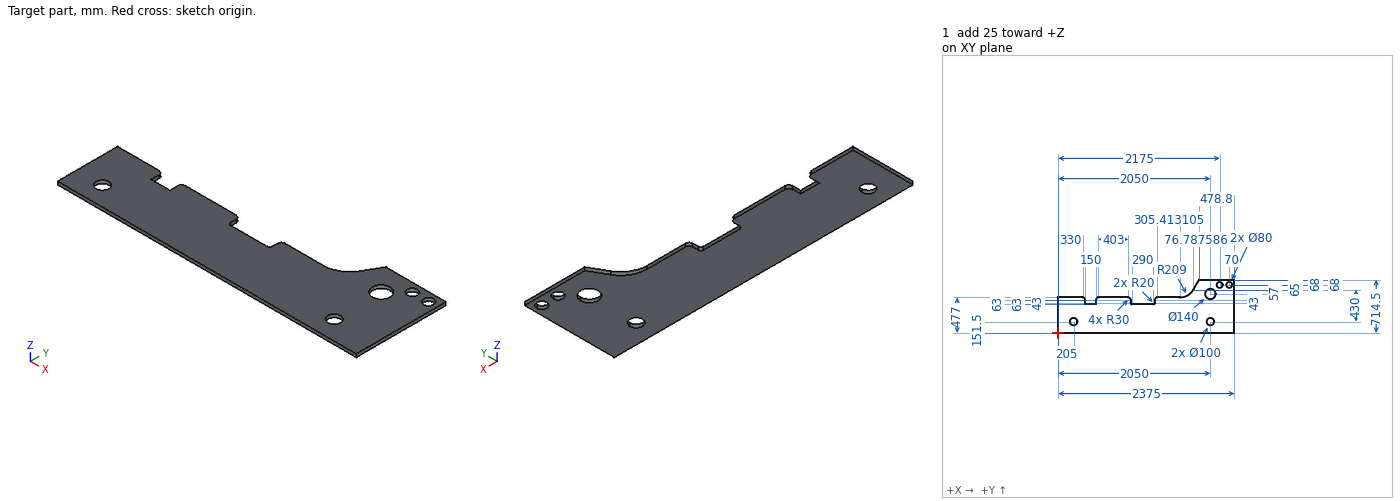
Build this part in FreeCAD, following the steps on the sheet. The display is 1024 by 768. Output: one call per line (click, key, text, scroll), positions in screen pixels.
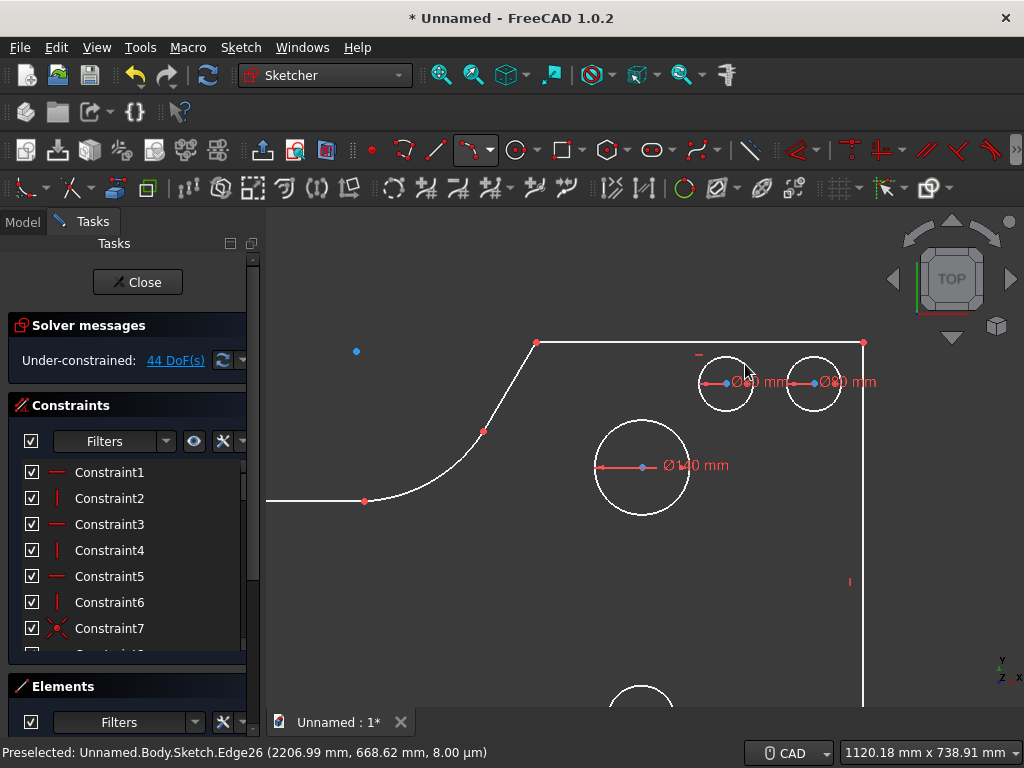
click(302, 501)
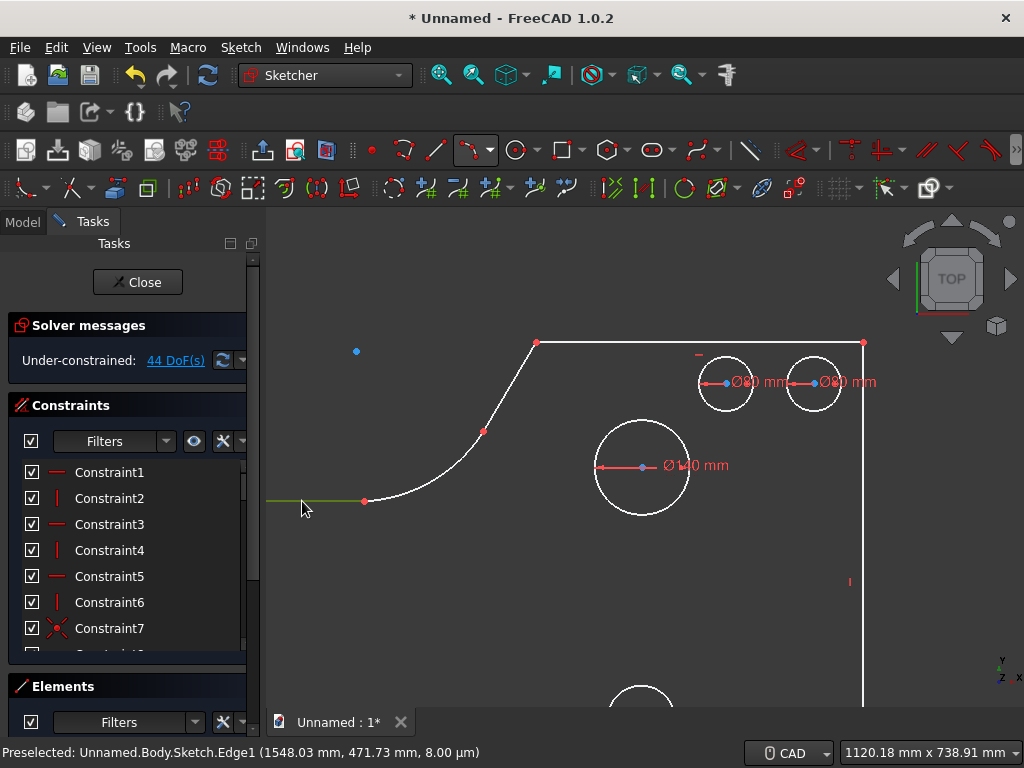
scroll(746, 417, down, 7)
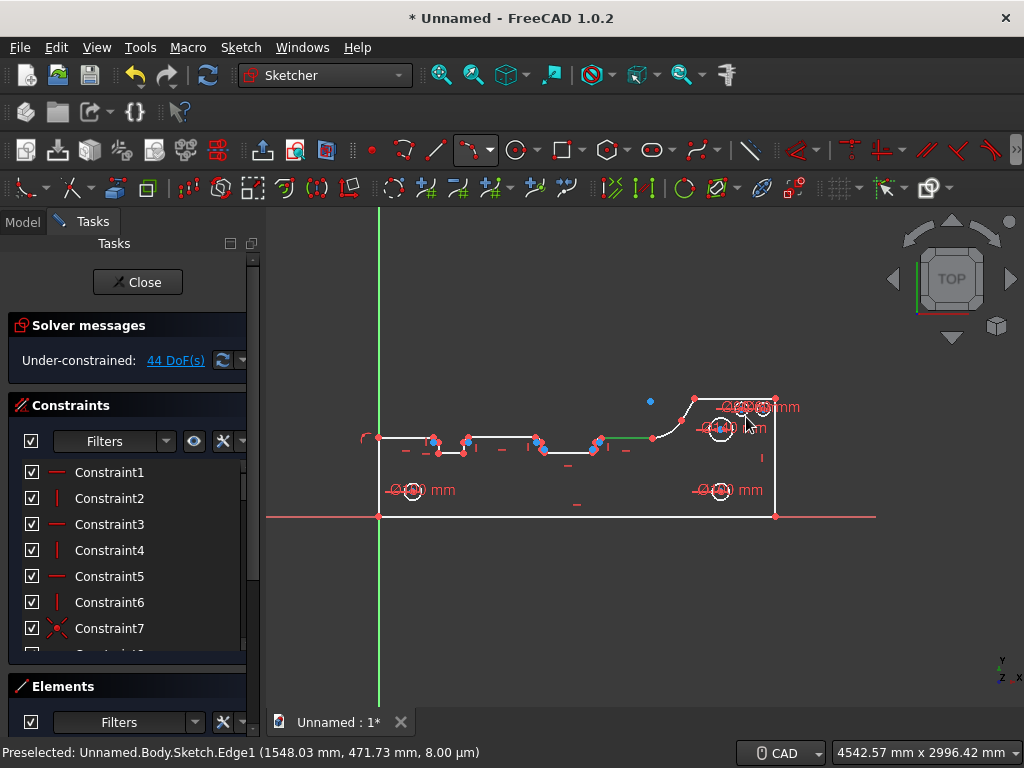
scroll(599, 438, up, 9)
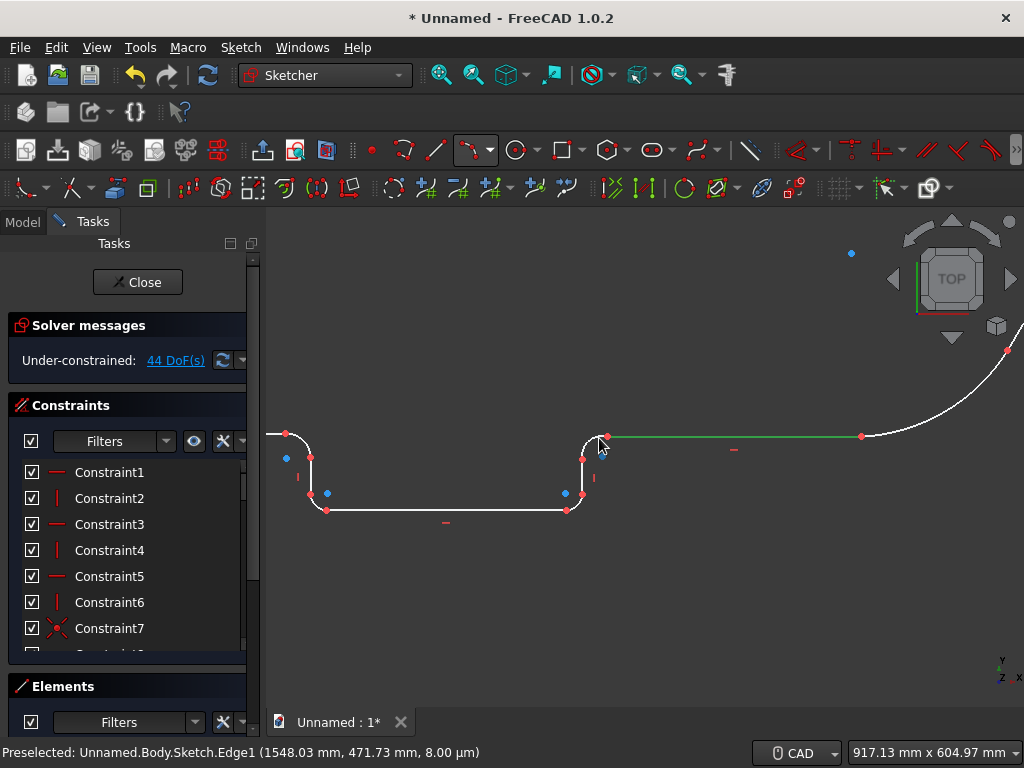
click(595, 437)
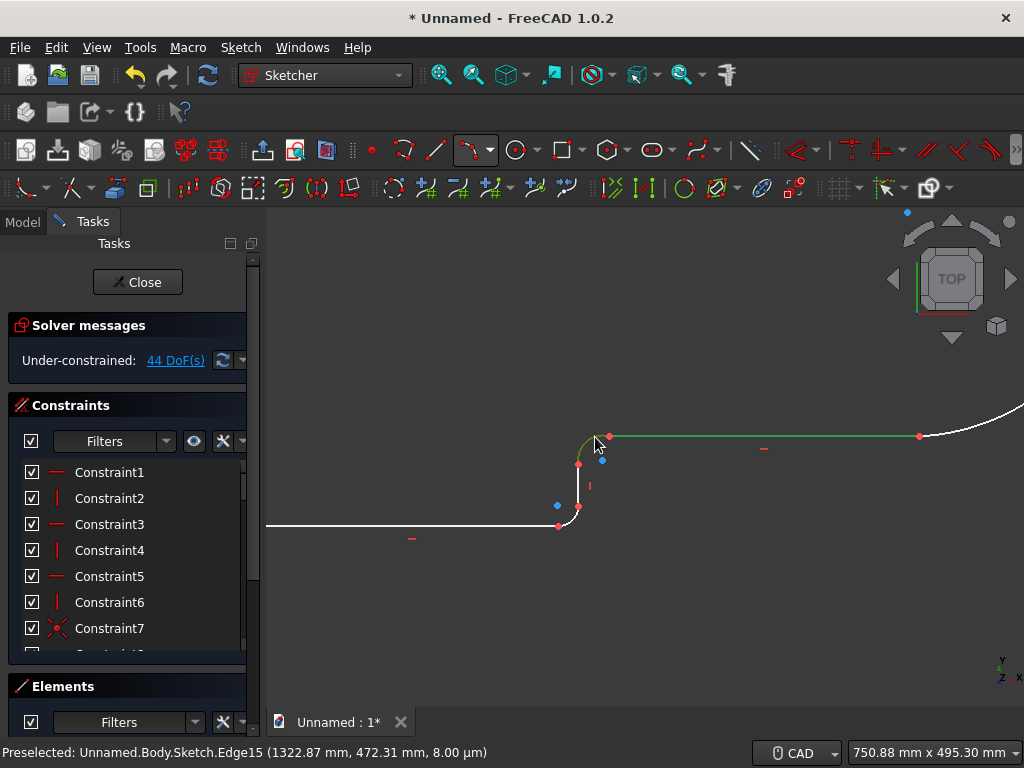
click(992, 150)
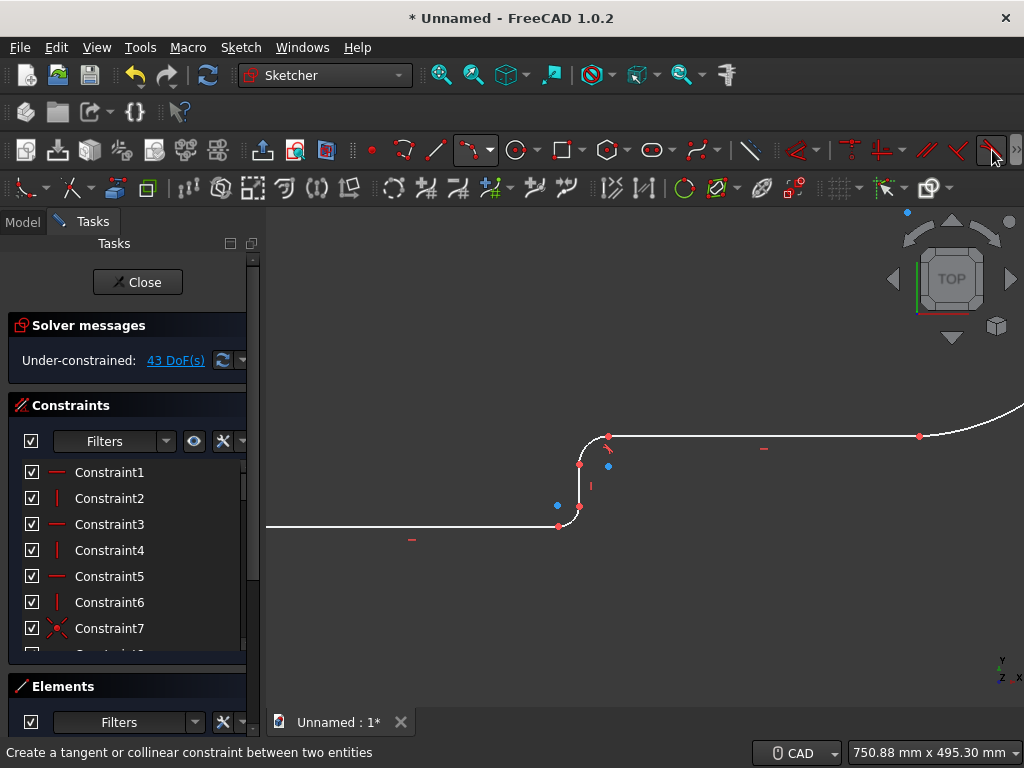
click(579, 477)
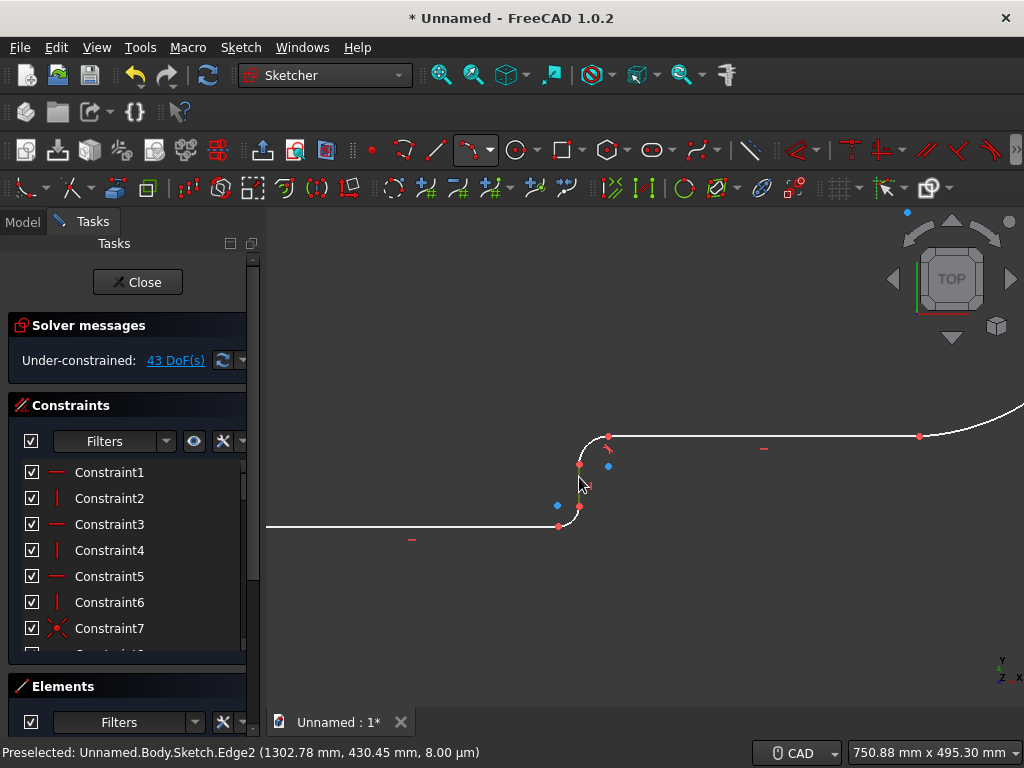
click(596, 439)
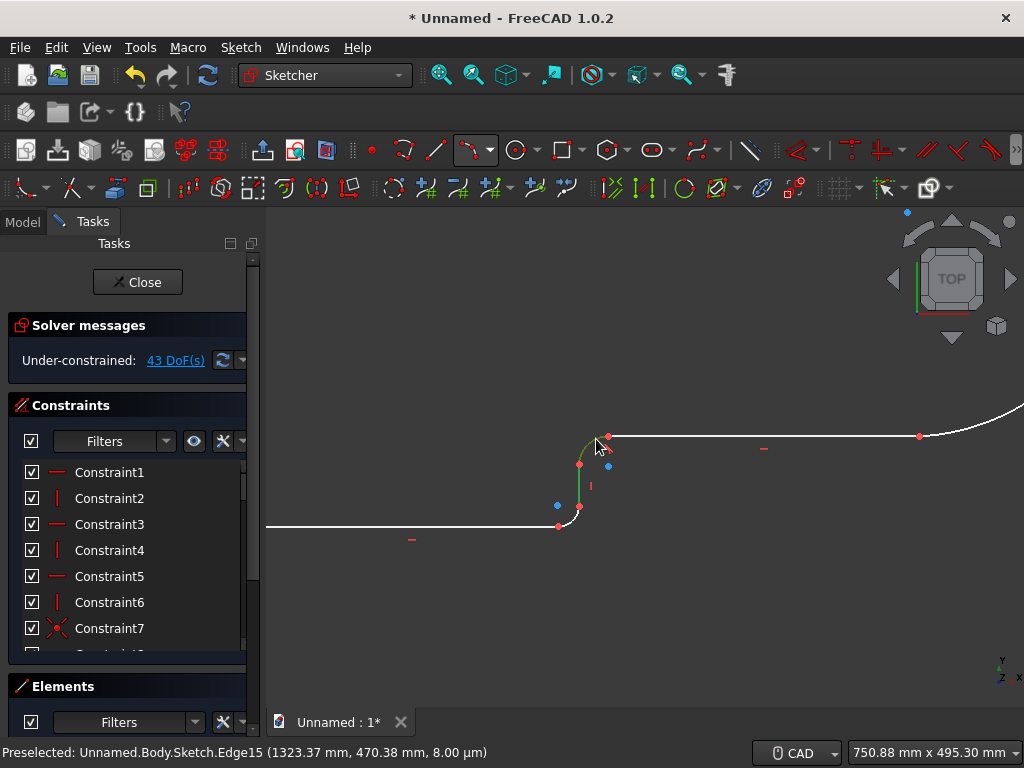
click(992, 150)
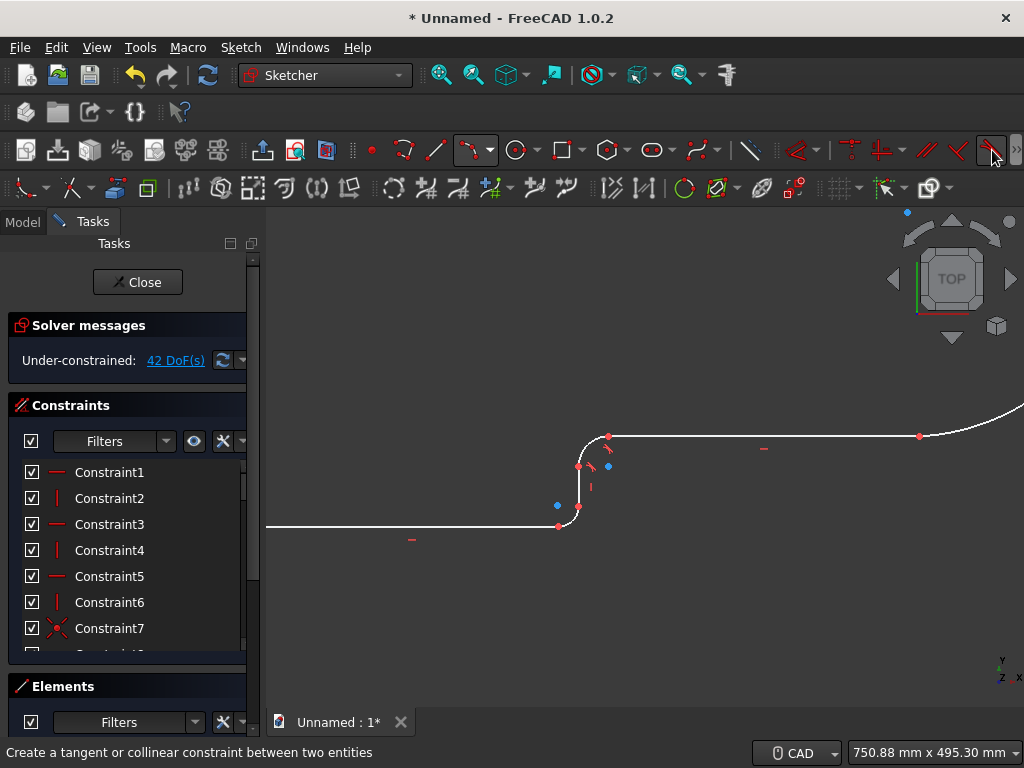
click(579, 478)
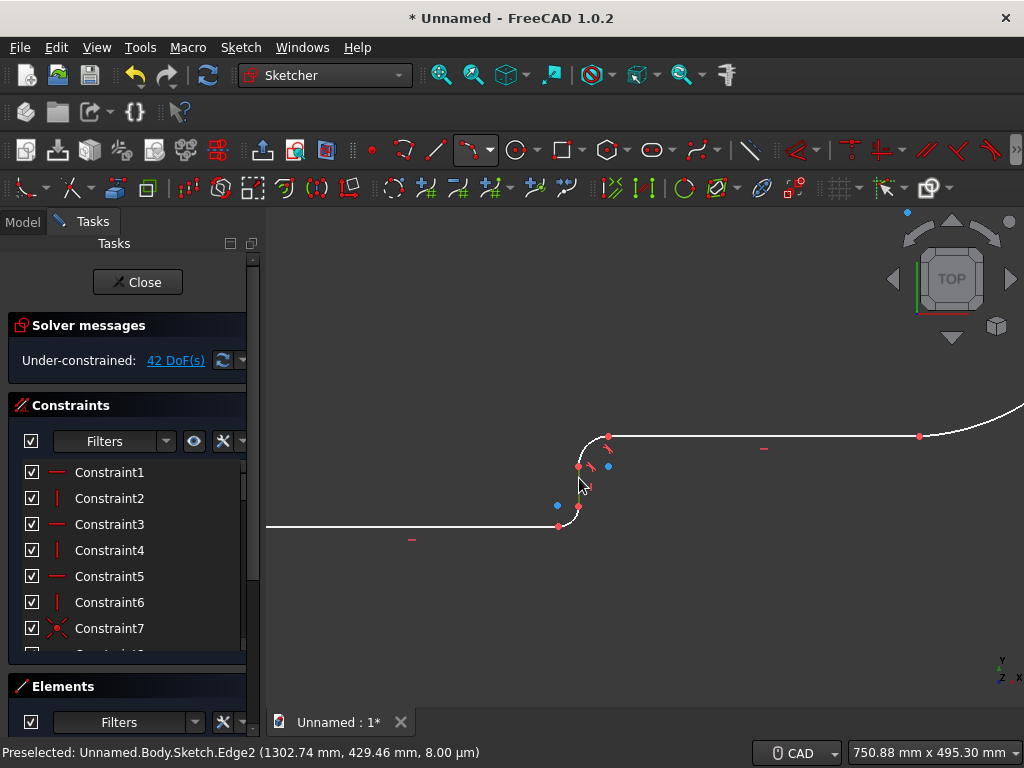
scroll(568, 524, up, 2)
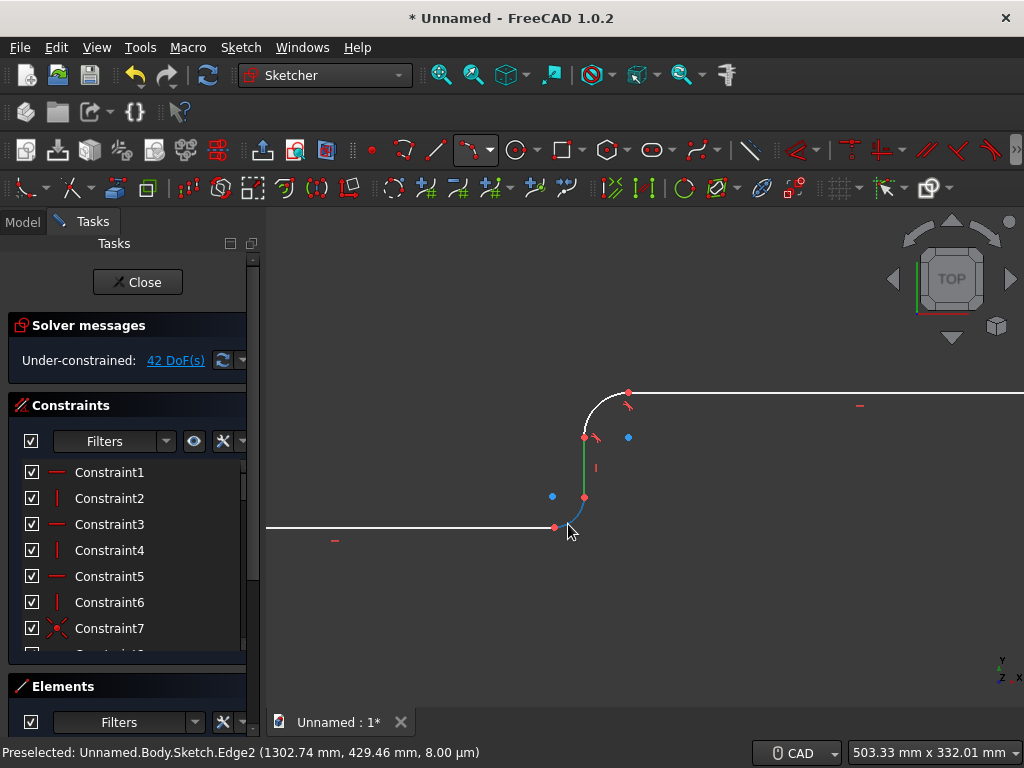
click(568, 524)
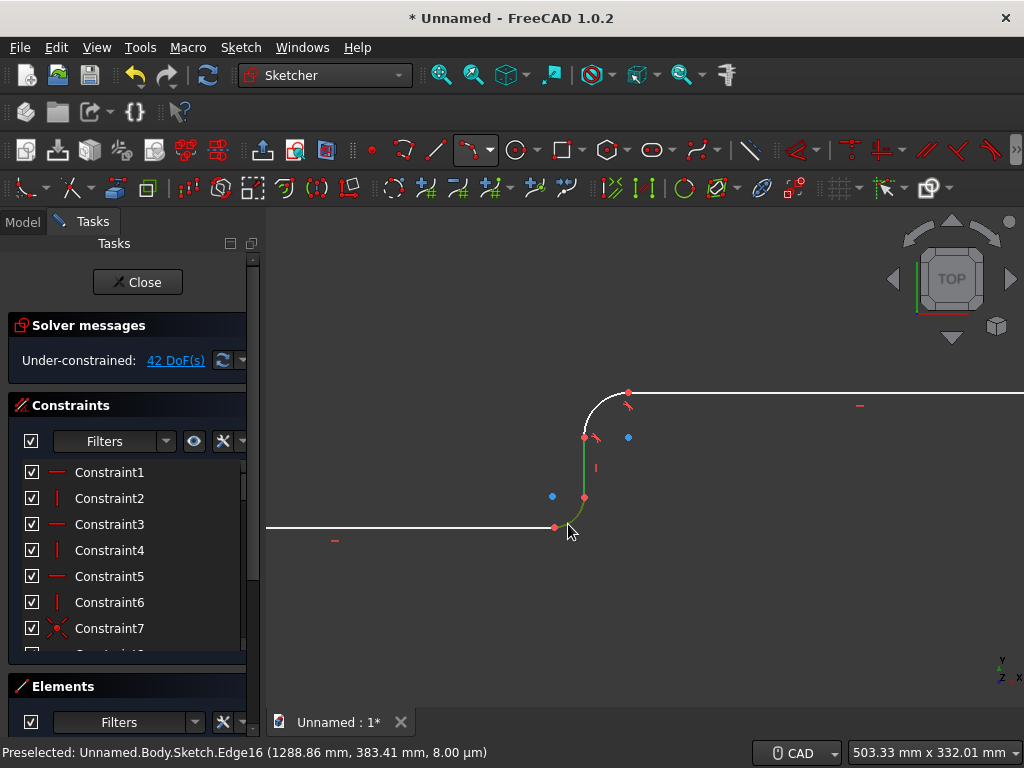
click(992, 150)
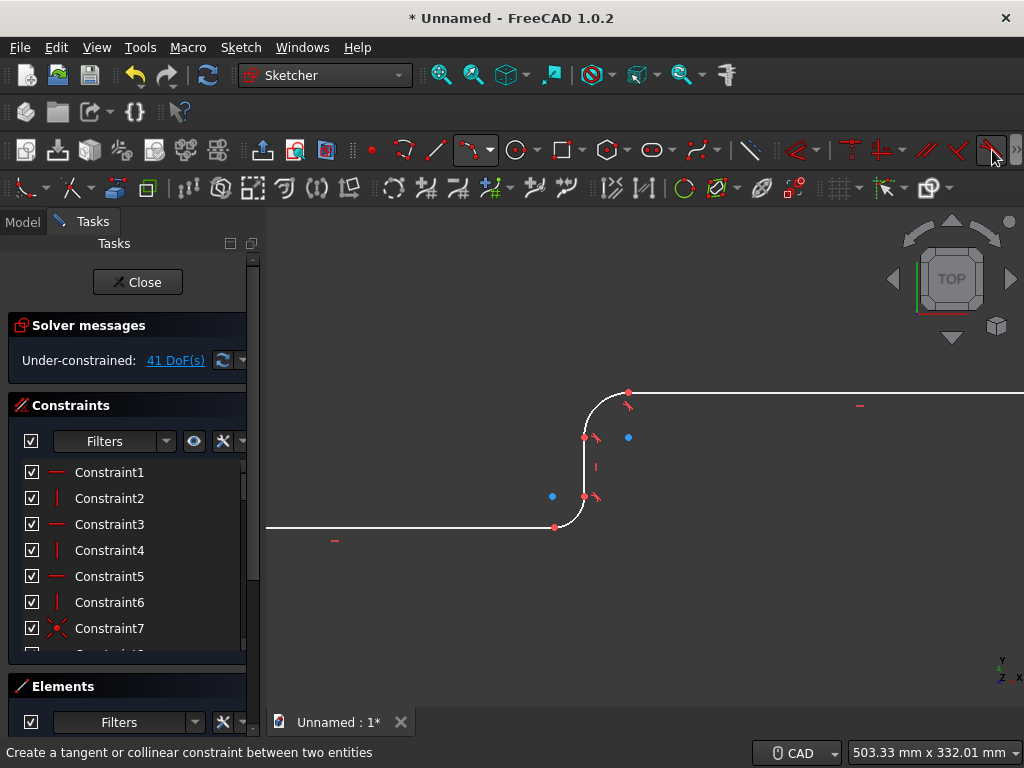
scroll(597, 444, down, 11)